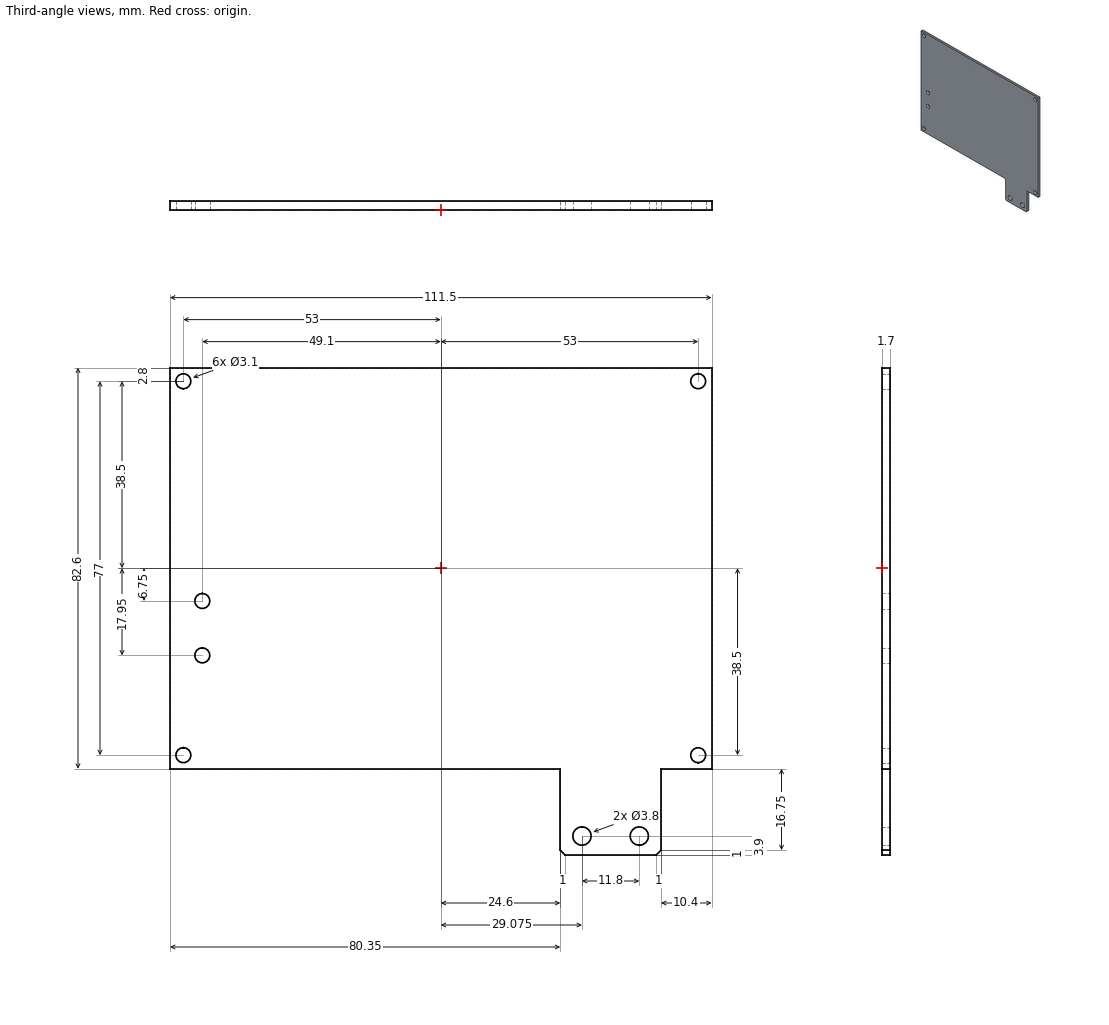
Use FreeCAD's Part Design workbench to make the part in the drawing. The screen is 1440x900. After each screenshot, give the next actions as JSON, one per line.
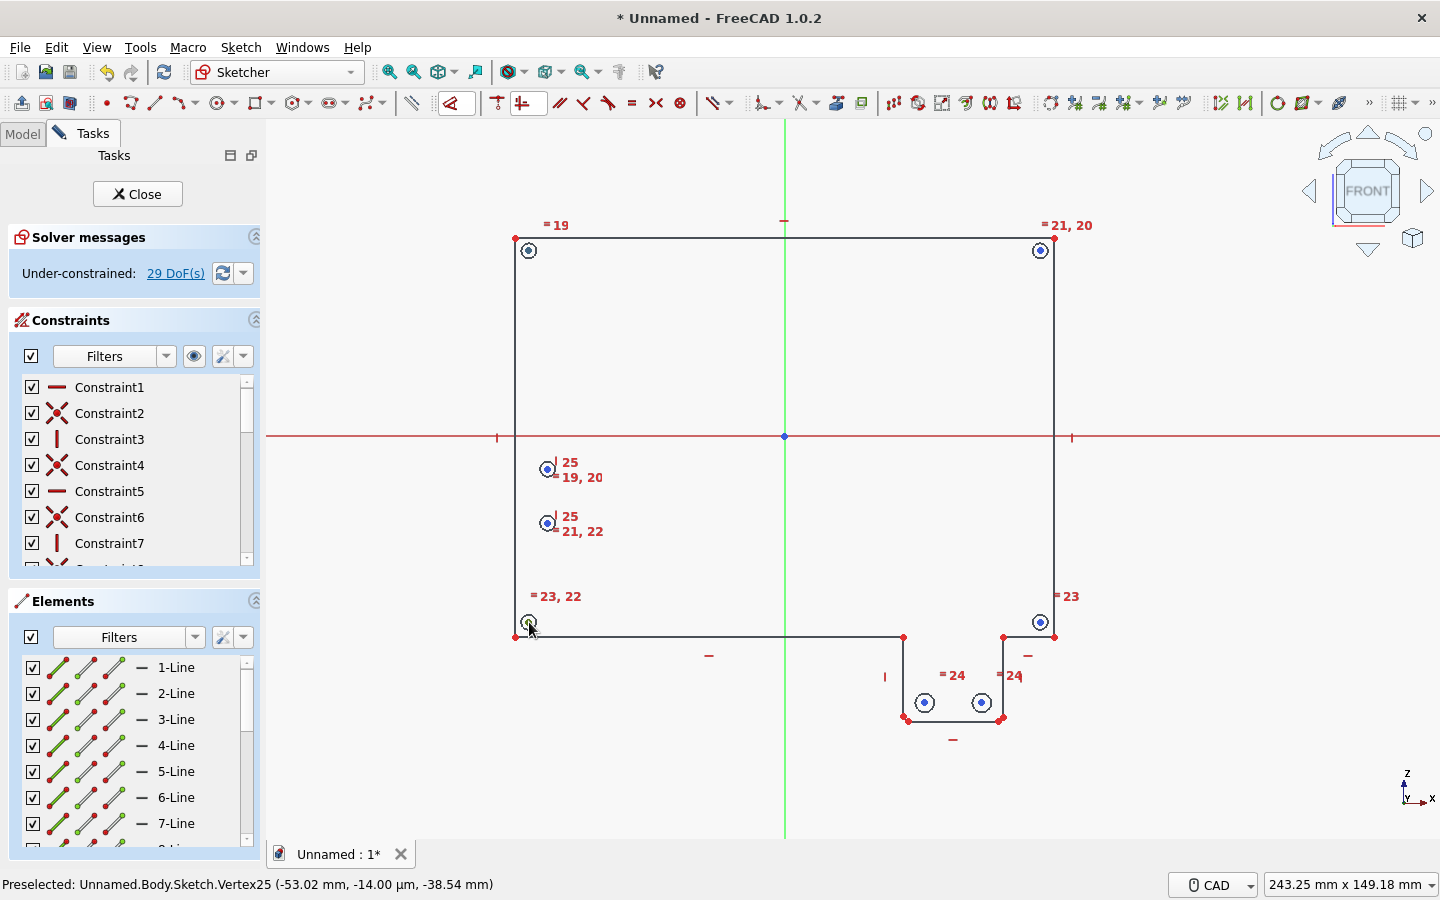
{"action": "key", "text": "v"}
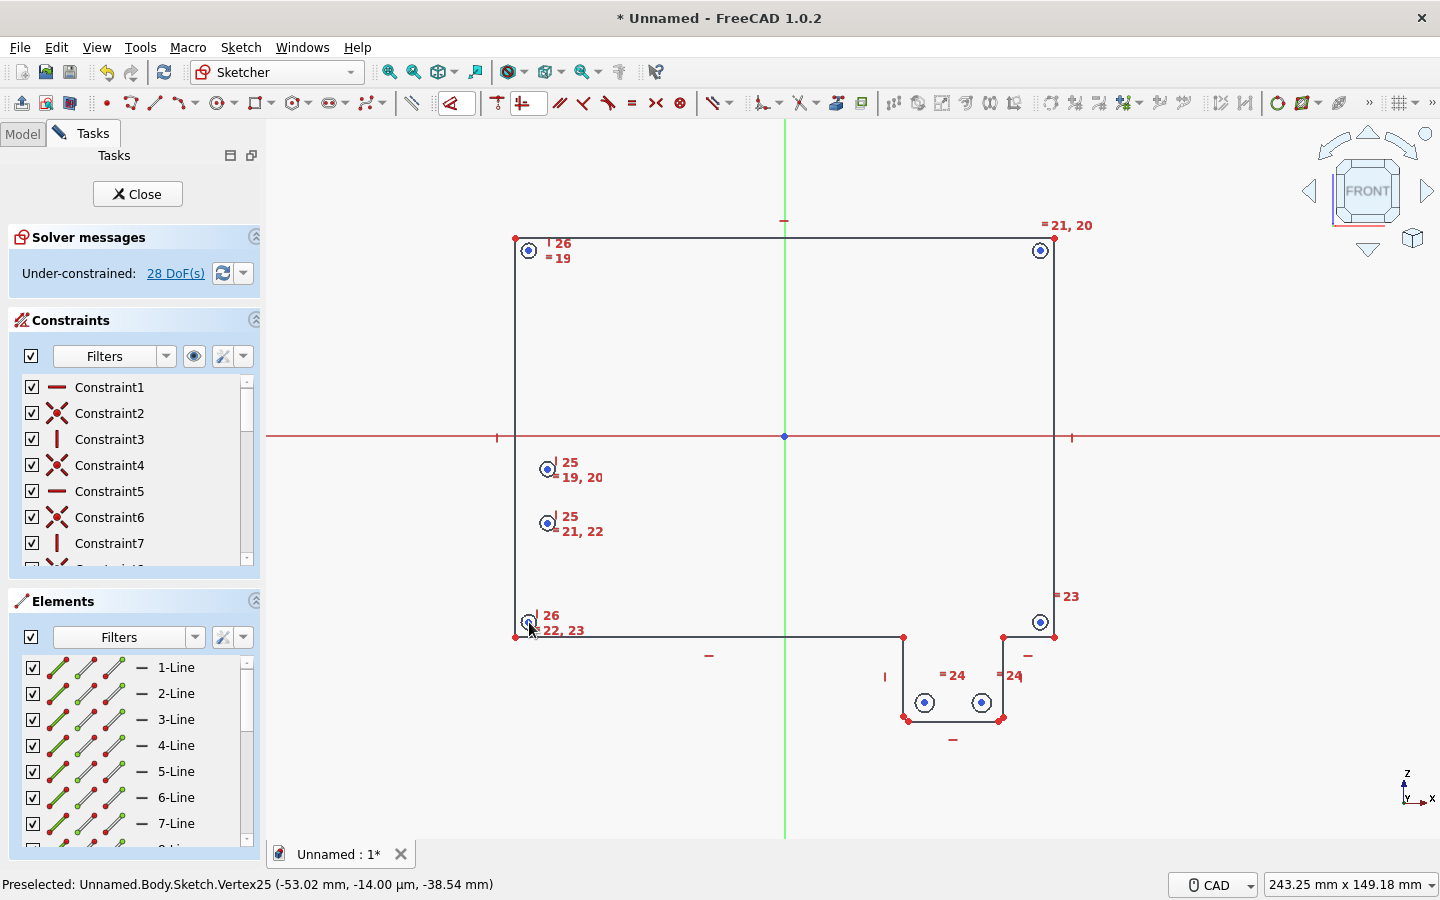
{"action": "left_click", "coordinate": [925, 703]}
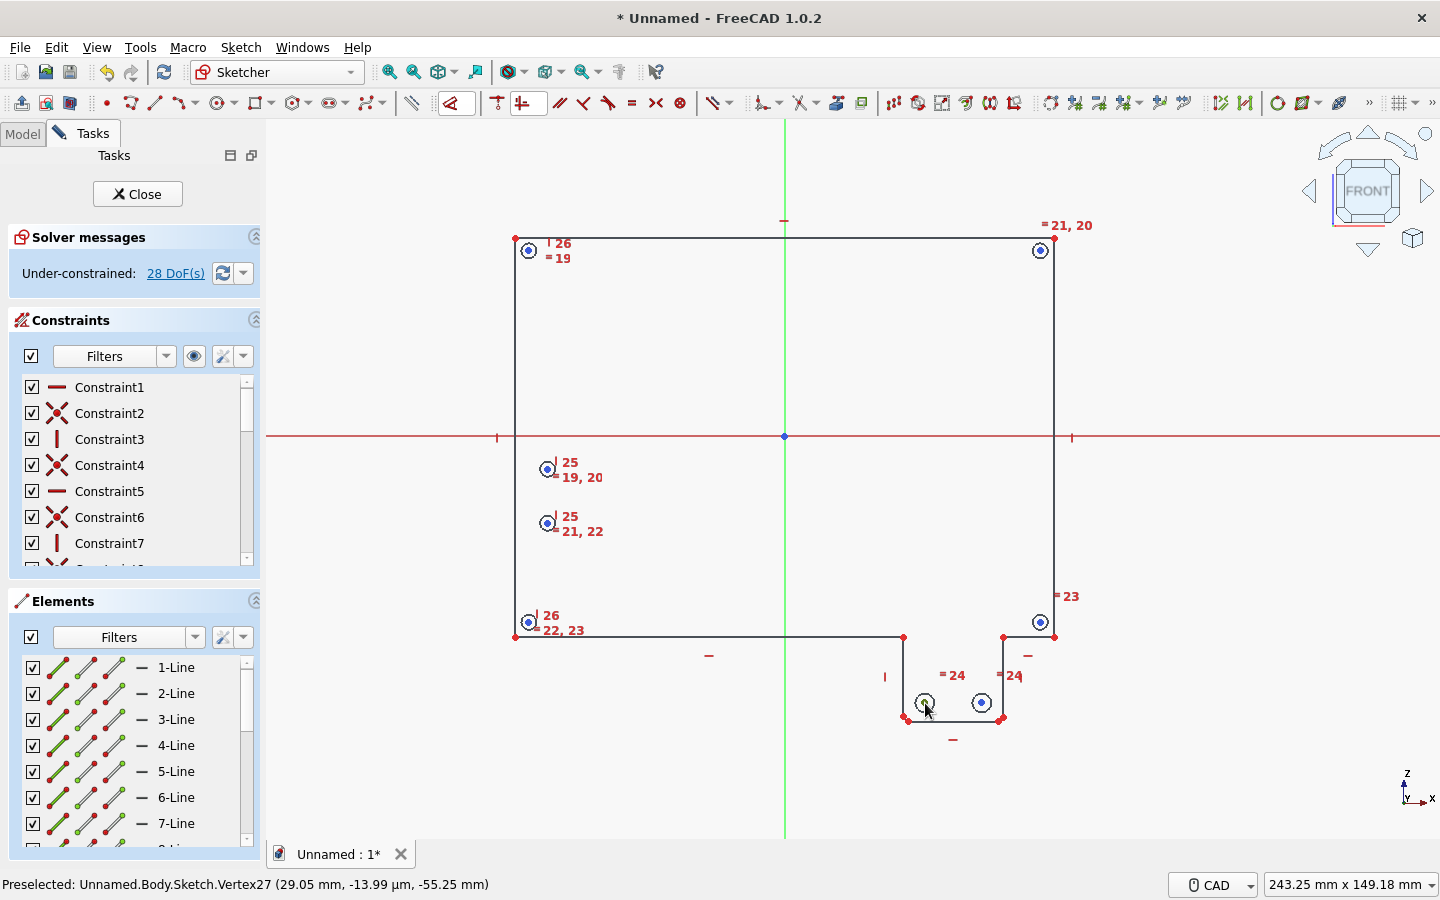
{"action": "left_click", "coordinate": [982, 703]}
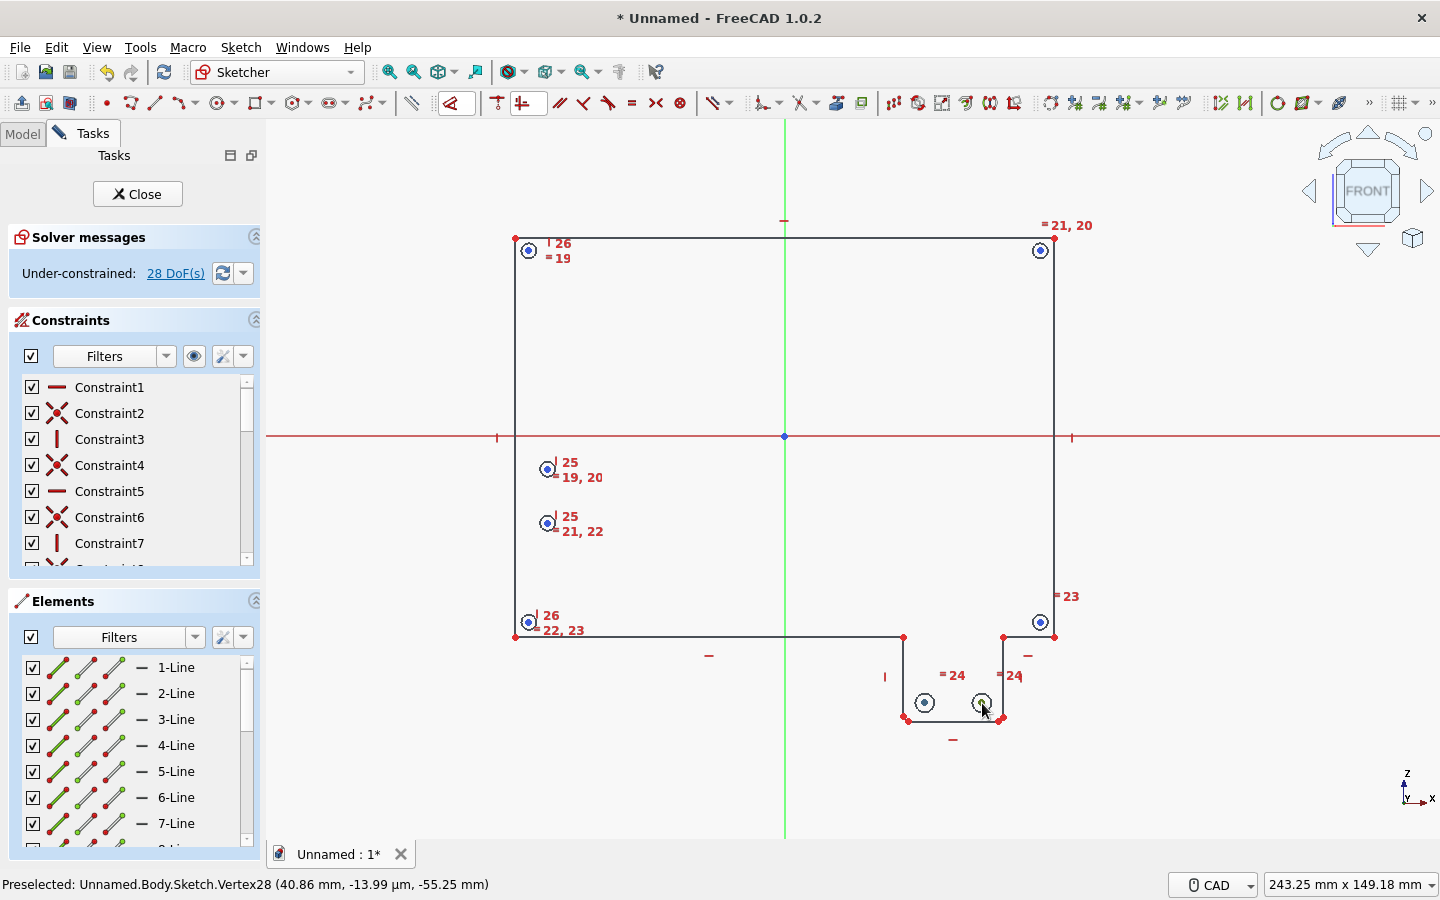
{"action": "key", "text": "h"}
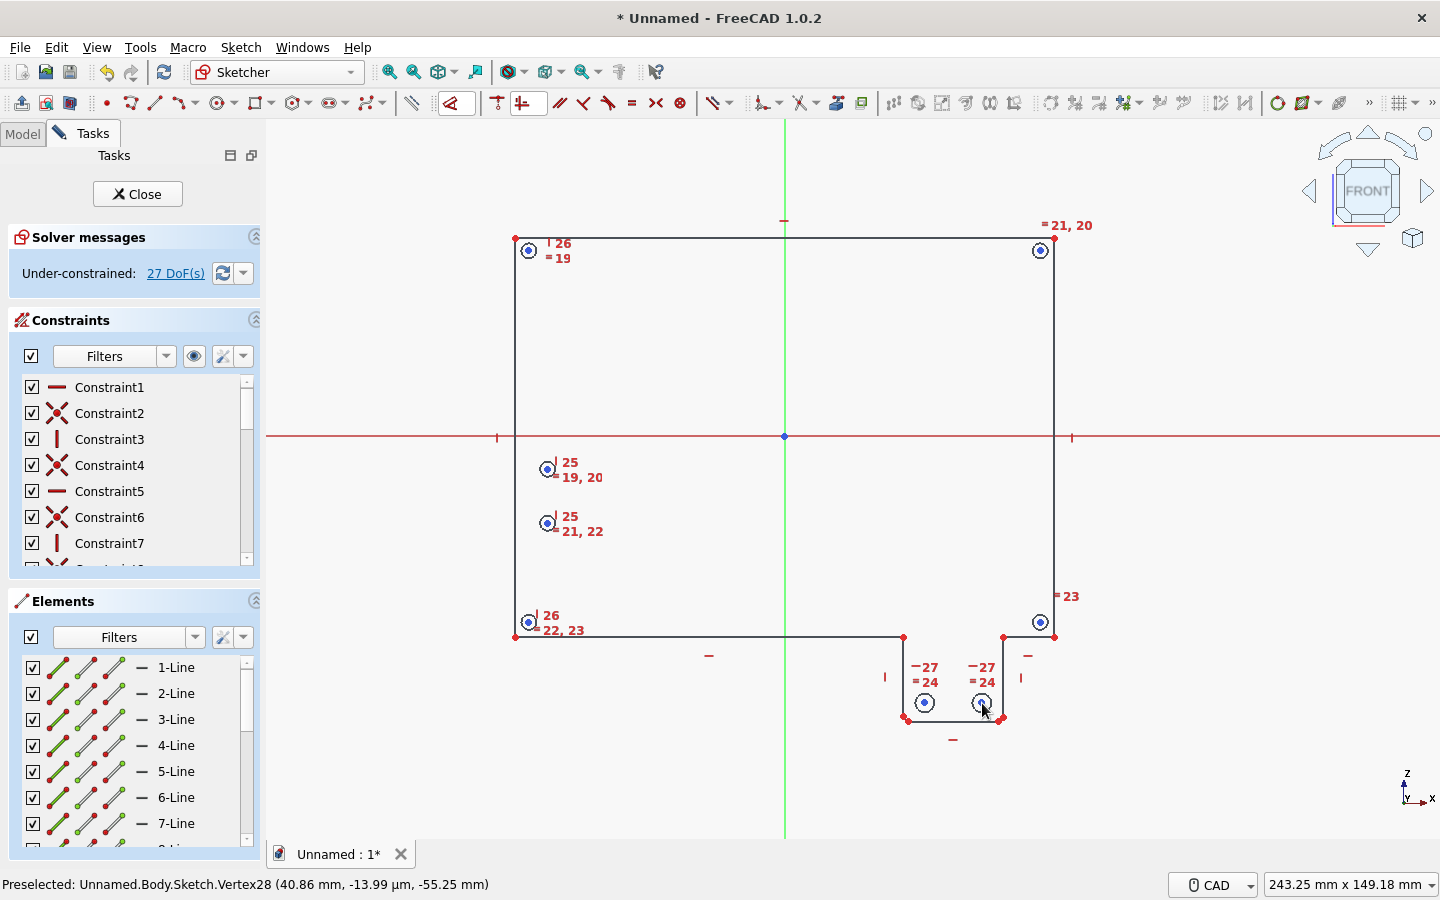
{"action": "scroll", "coordinate": [534, 246], "scroll_direction": "up", "scroll_amount": 5}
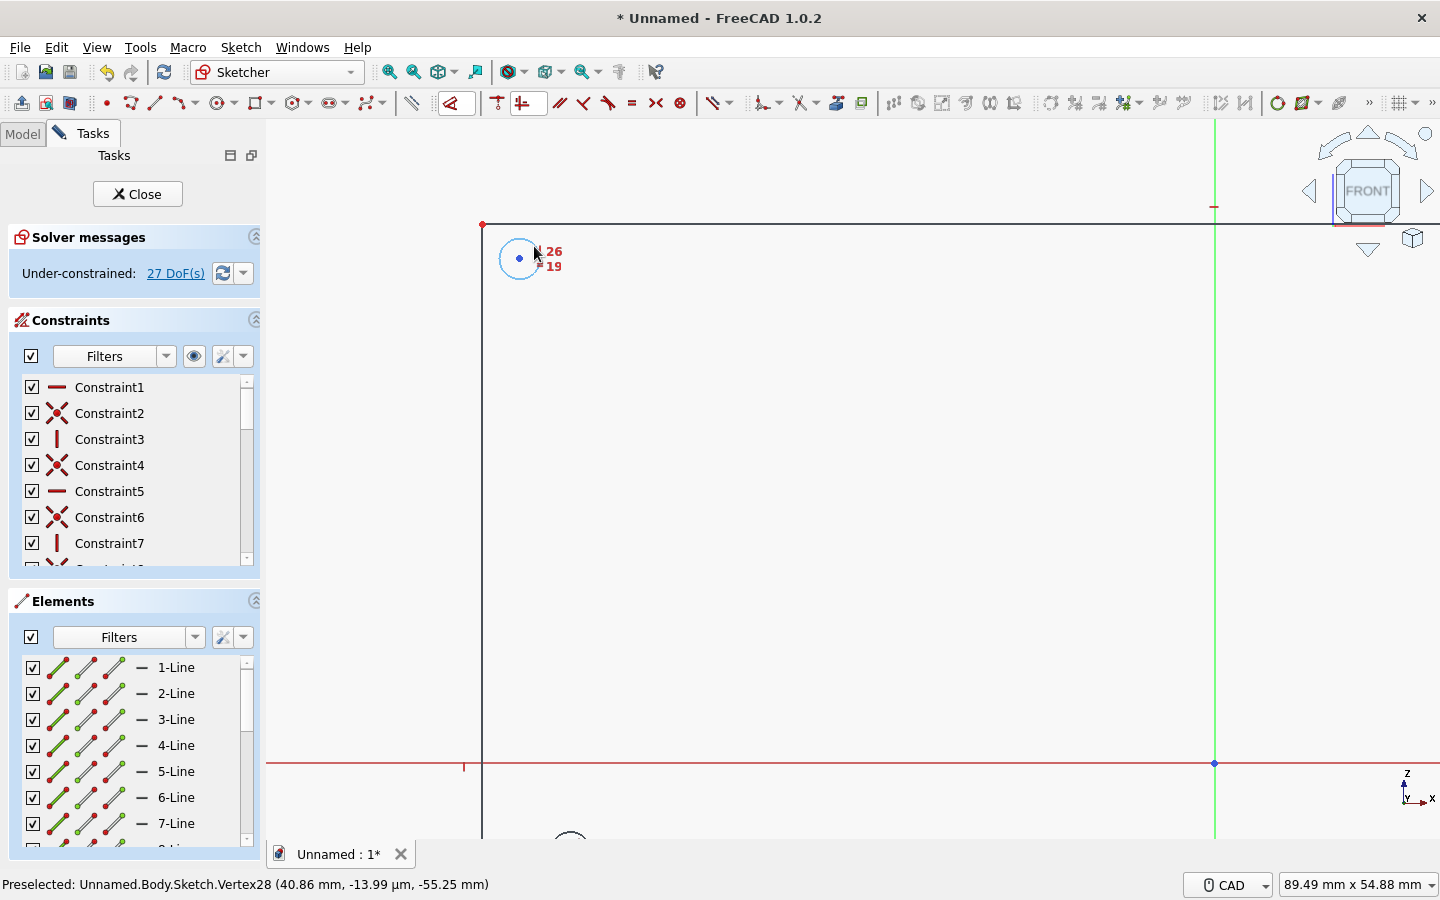
{"action": "left_click", "coordinate": [534, 245]}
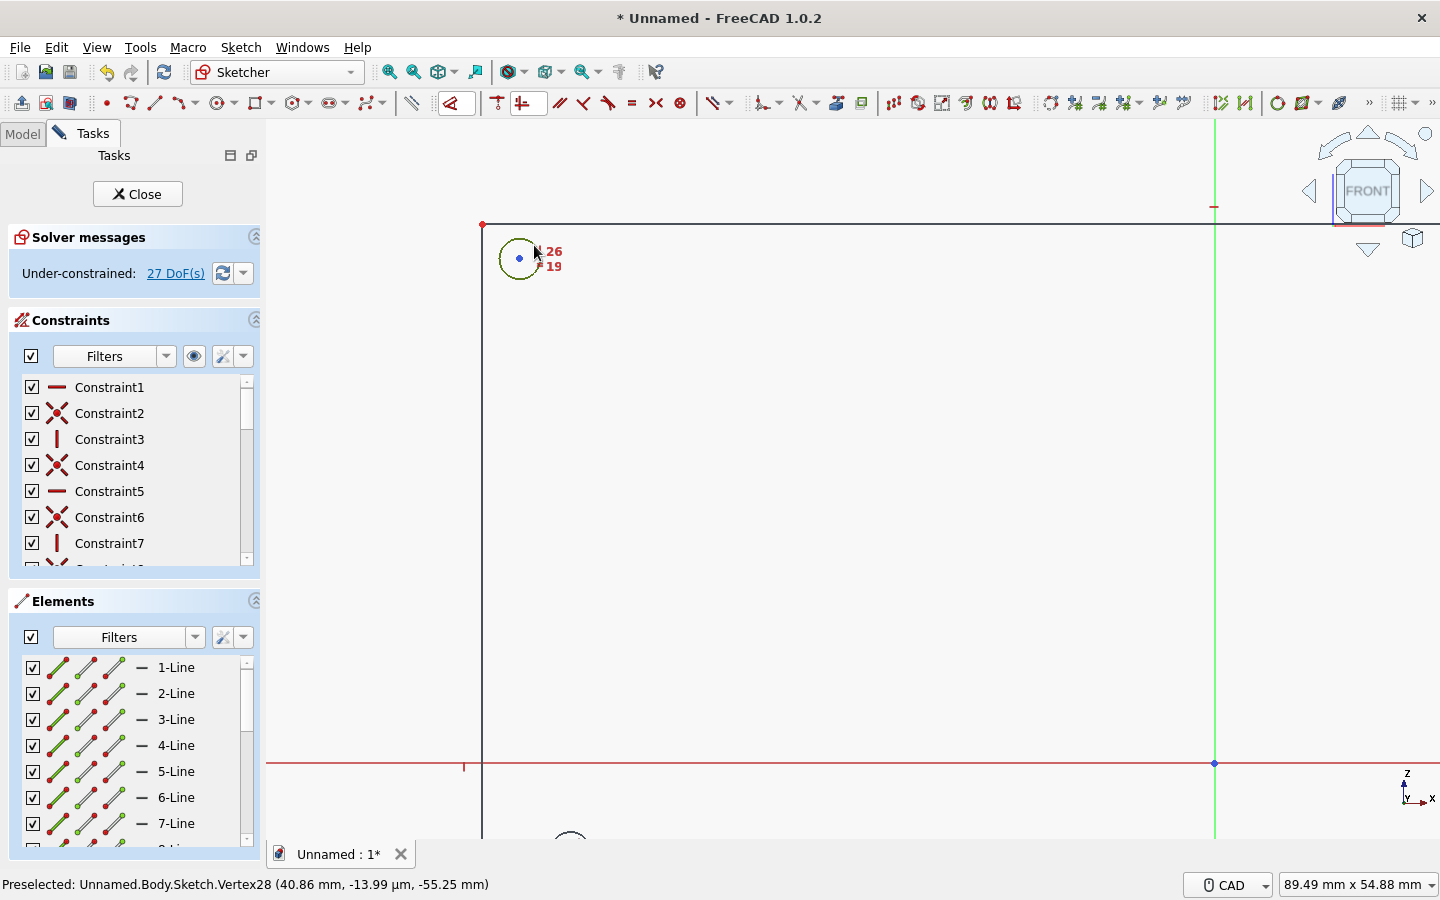
{"action": "key", "text": "k o"}